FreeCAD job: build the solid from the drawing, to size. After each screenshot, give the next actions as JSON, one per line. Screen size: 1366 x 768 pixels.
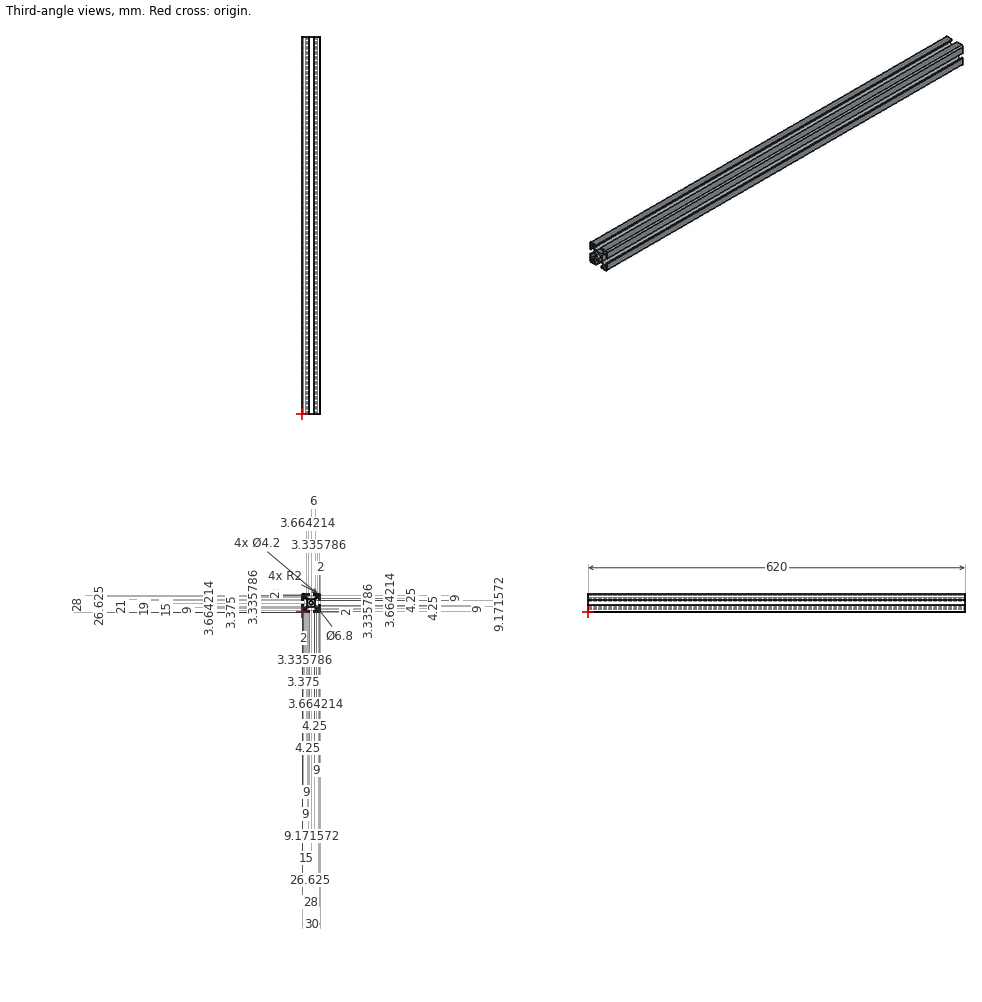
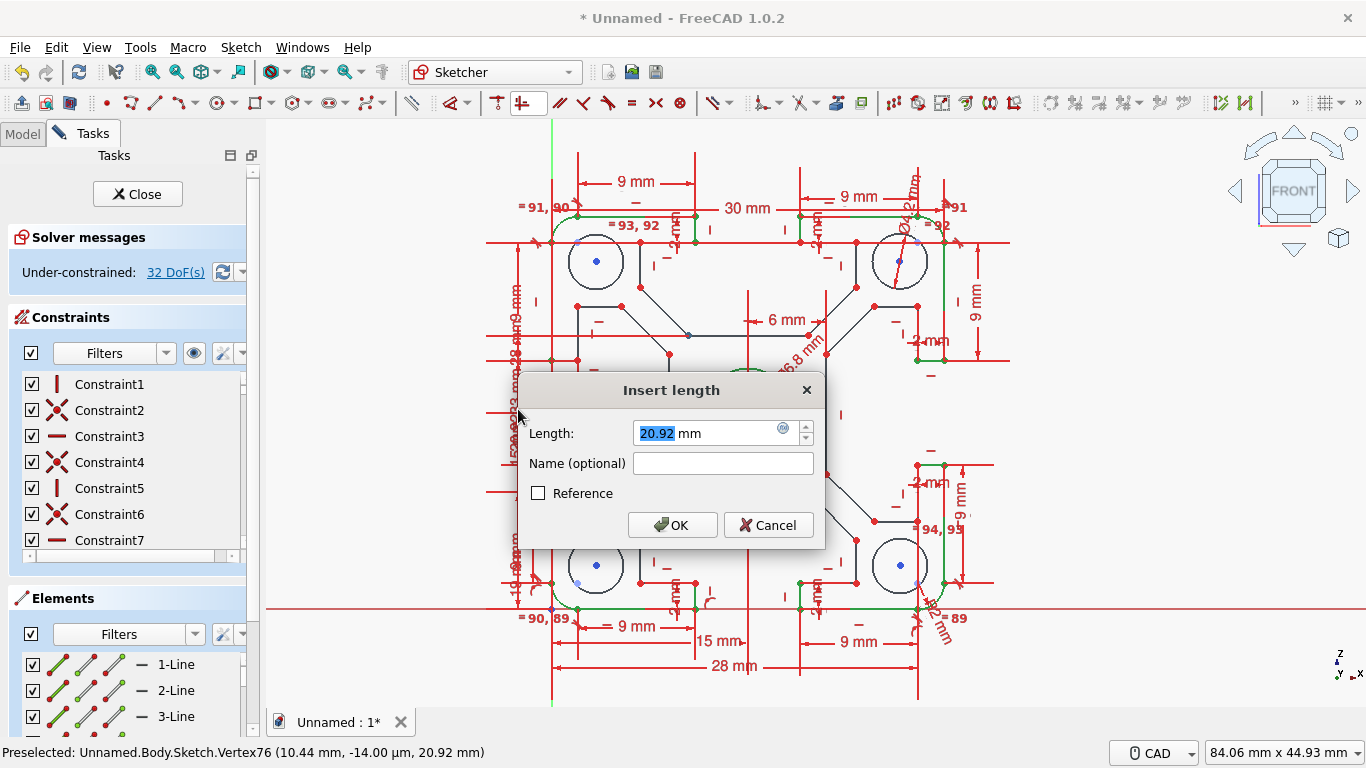
{"action": "type", "text": "21"}
{"action": "key", "text": "Return"}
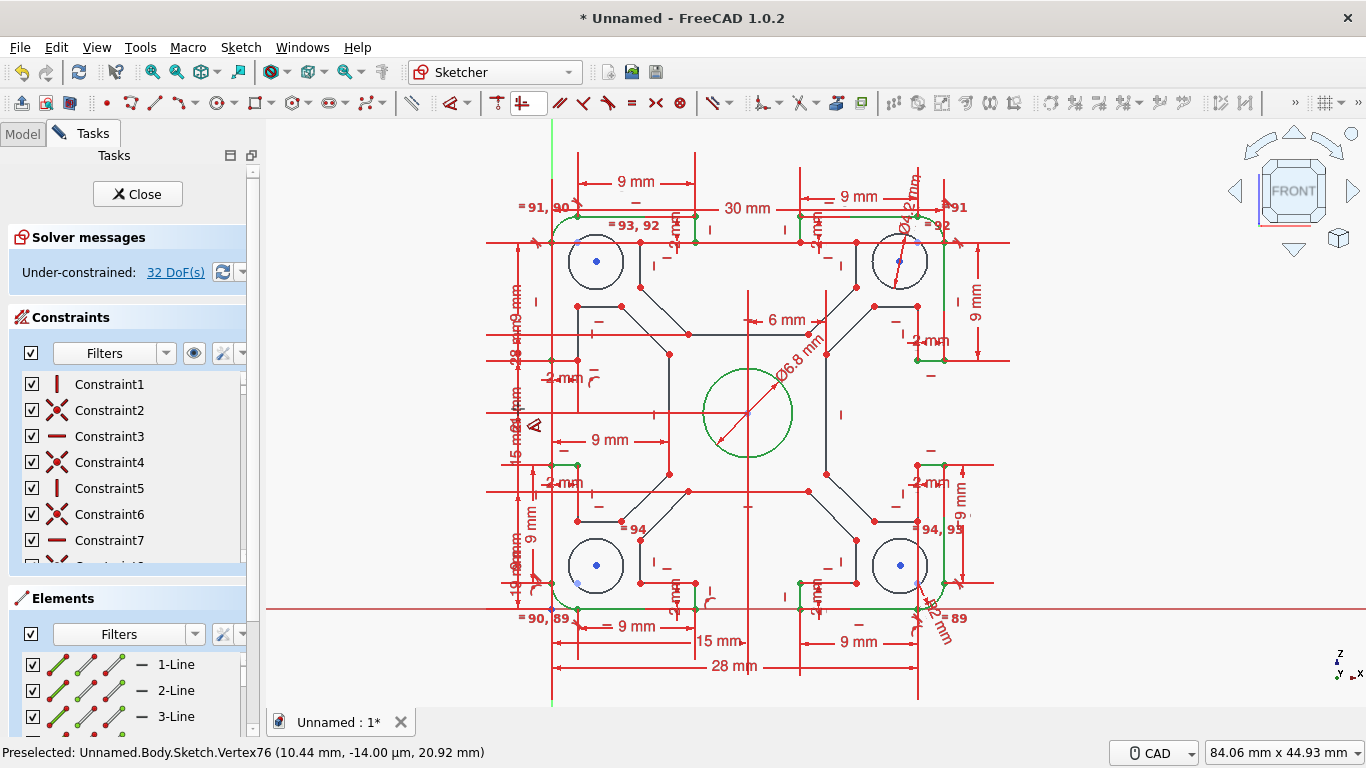
{"action": "left_click", "coordinate": [918, 344]}
{"action": "left_click", "coordinate": [884, 321]}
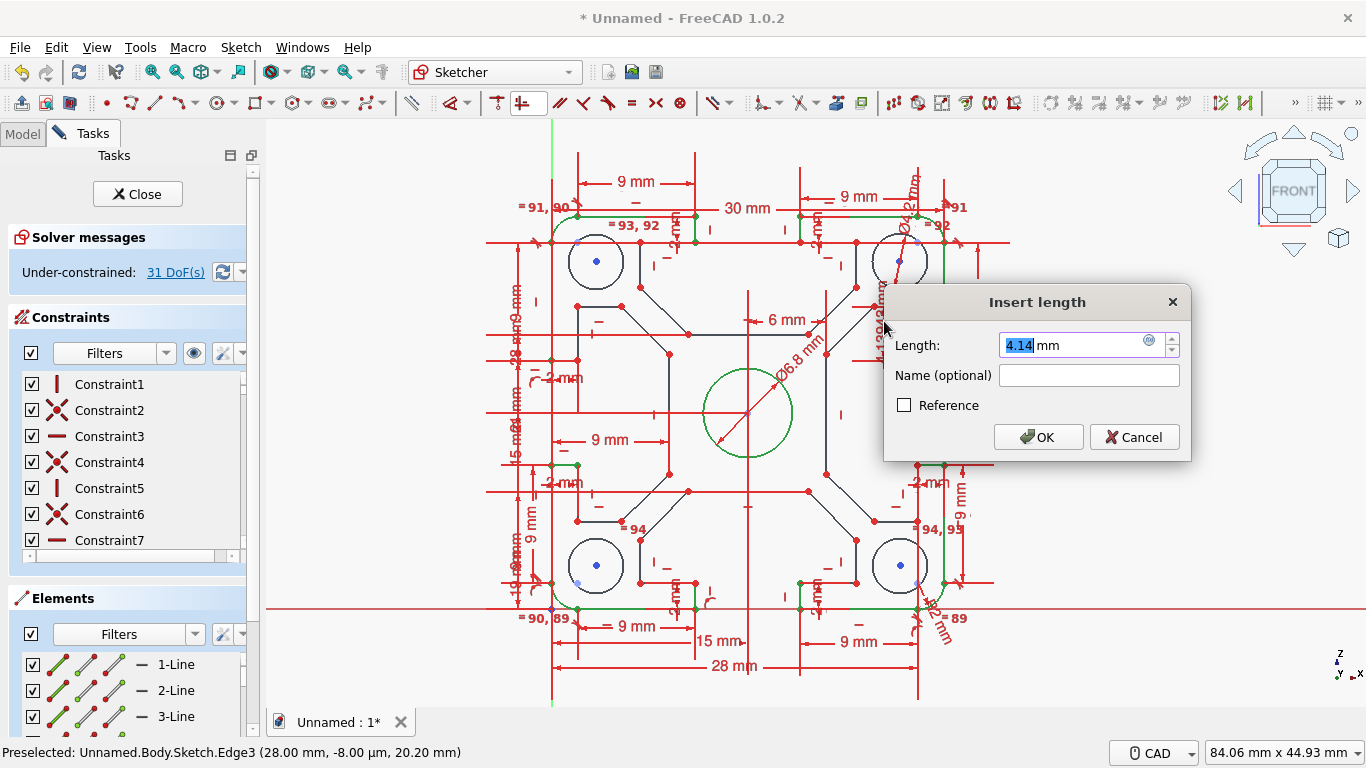
{"action": "type", "text": "4.25"}
{"action": "key", "text": "Return"}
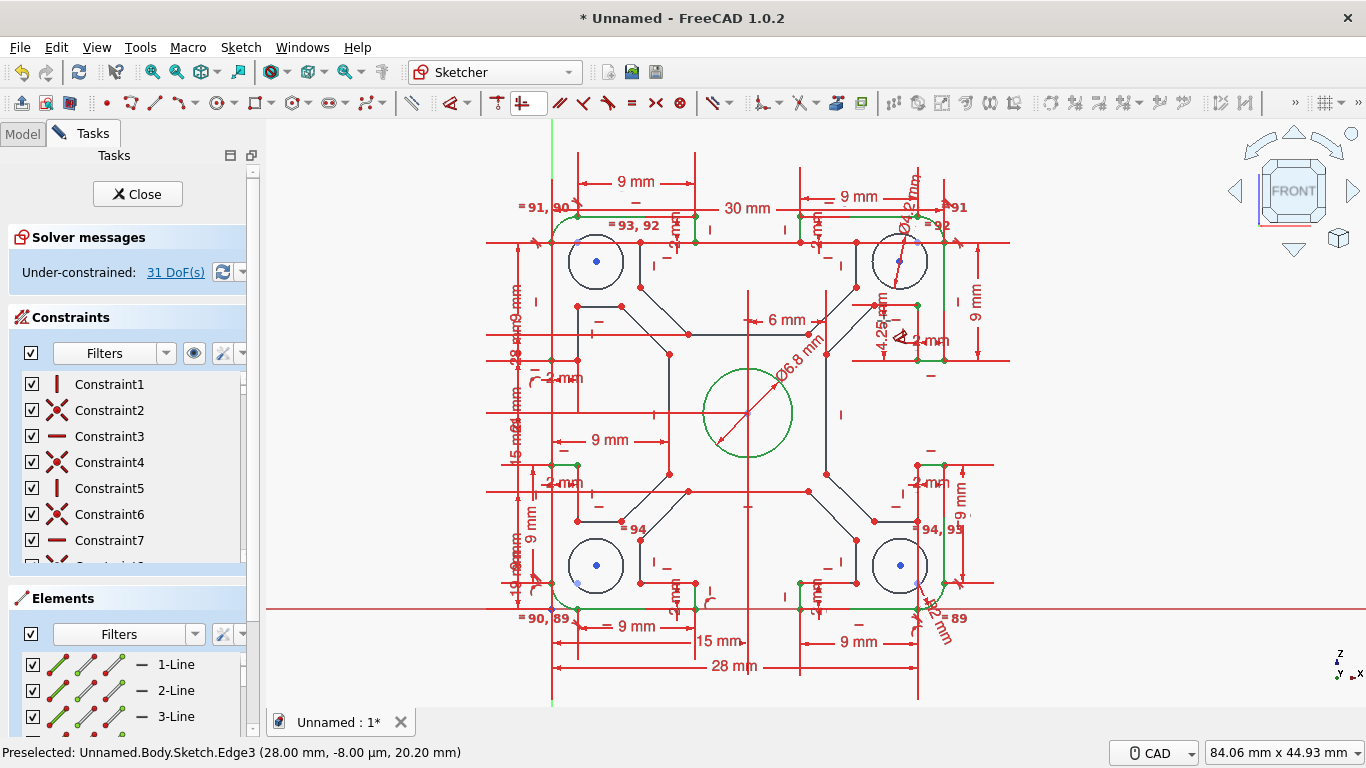
{"action": "left_click", "coordinate": [918, 505]}
{"action": "left_click", "coordinate": [884, 506]}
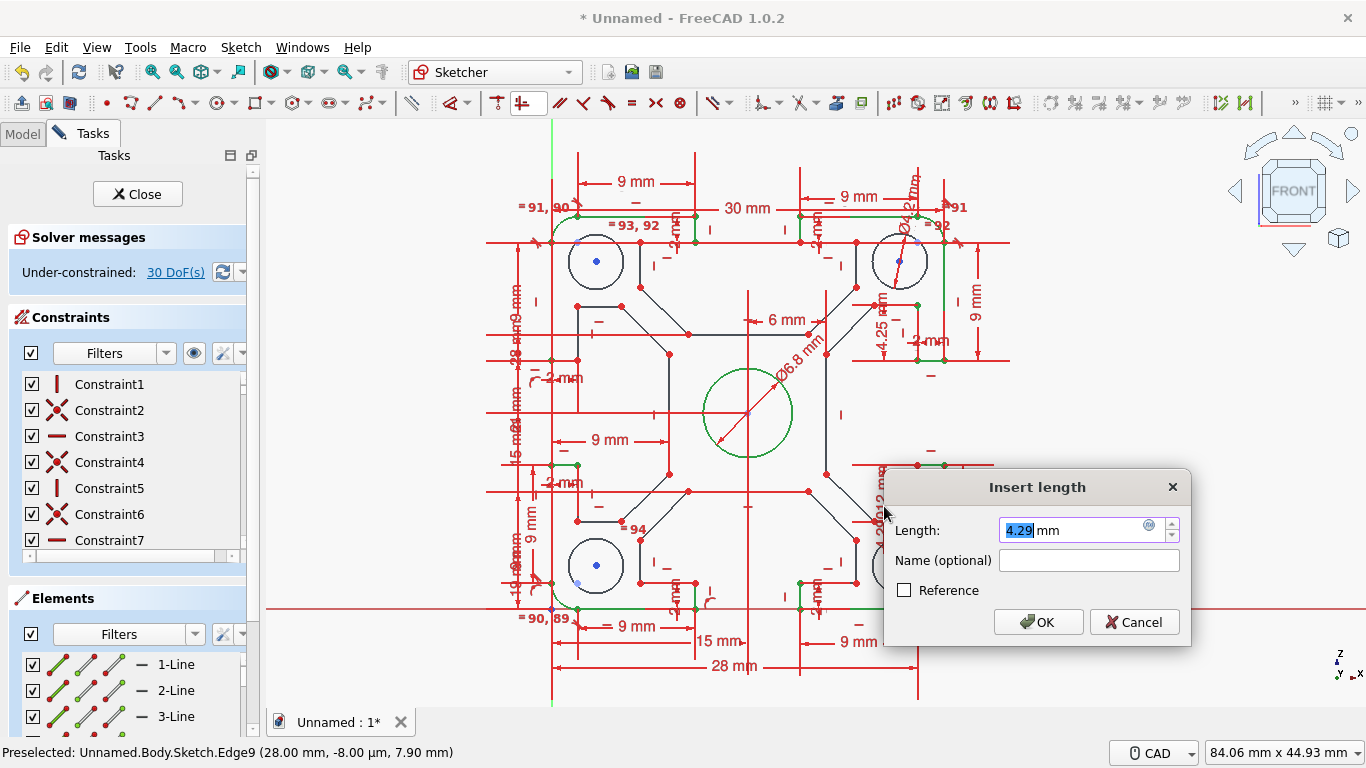
{"action": "type", "text": "4.25"}
{"action": "key", "text": "Return"}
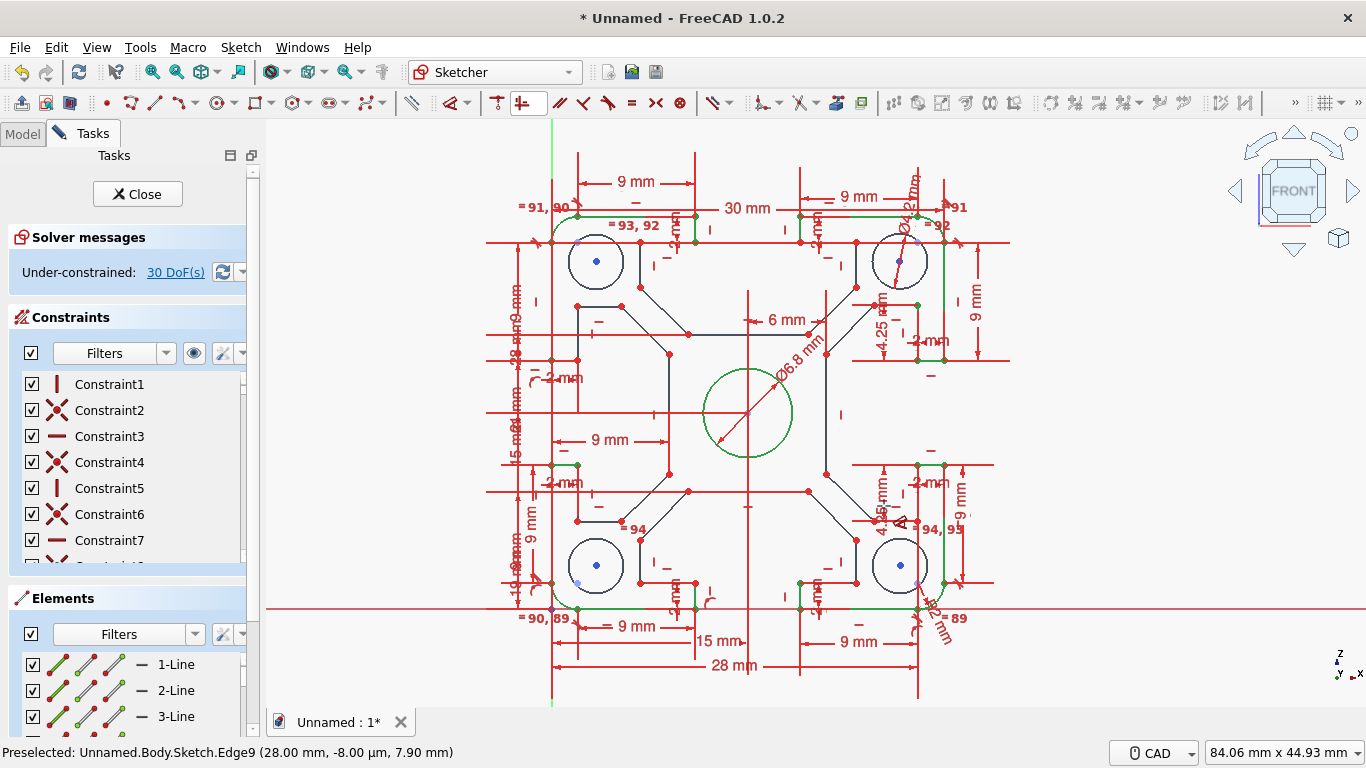
{"action": "left_click", "coordinate": [817, 583]}
{"action": "left_click", "coordinate": [828, 549]}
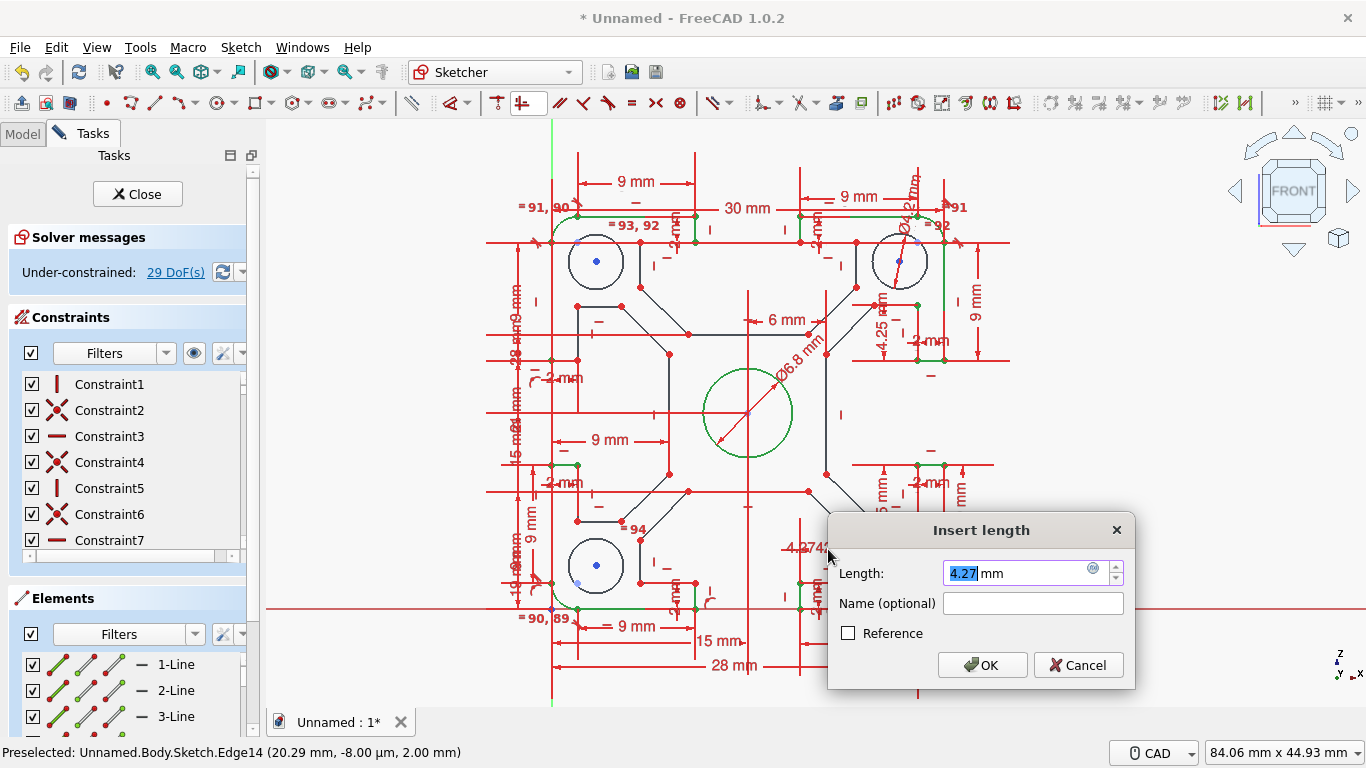
{"action": "type", "text": "4.25"}
{"action": "key", "text": "Return"}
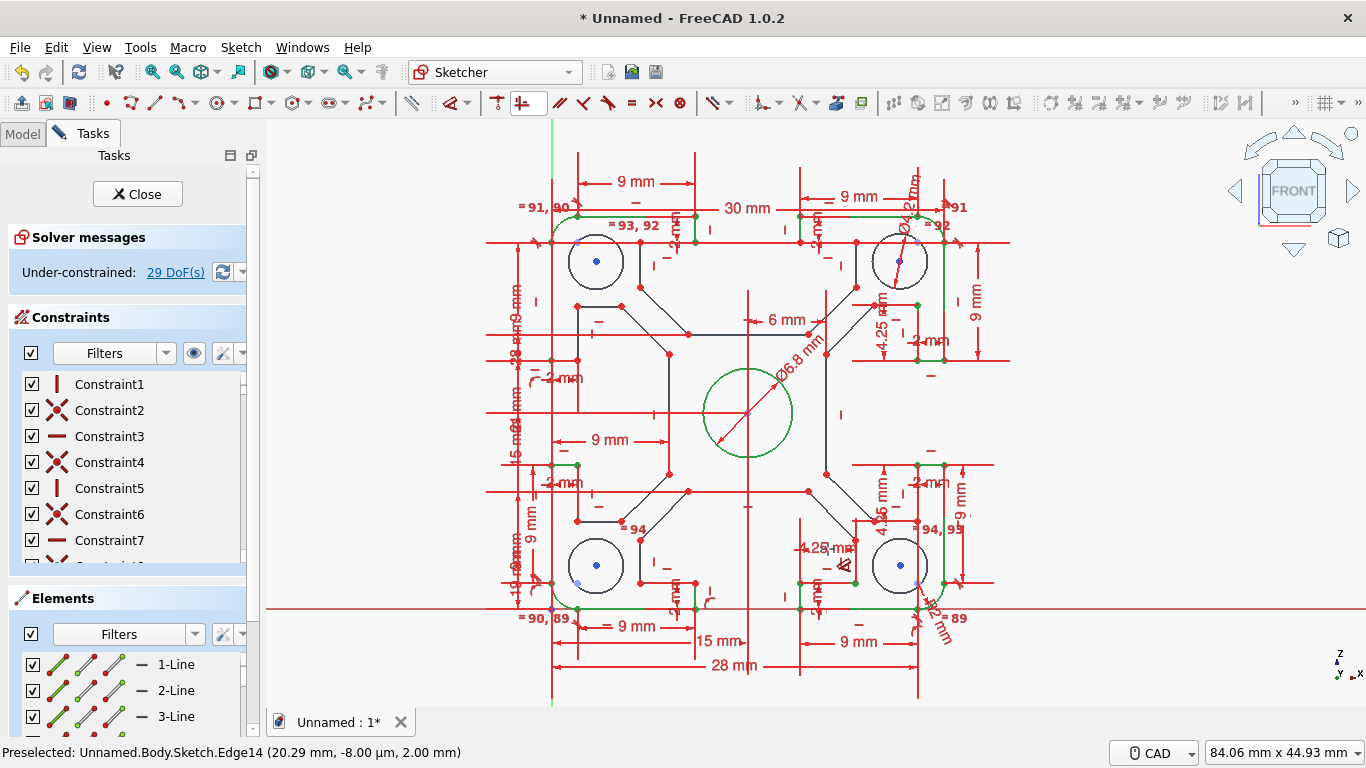
{"action": "left_click", "coordinate": [657, 583]}
{"action": "left_click", "coordinate": [668, 549]}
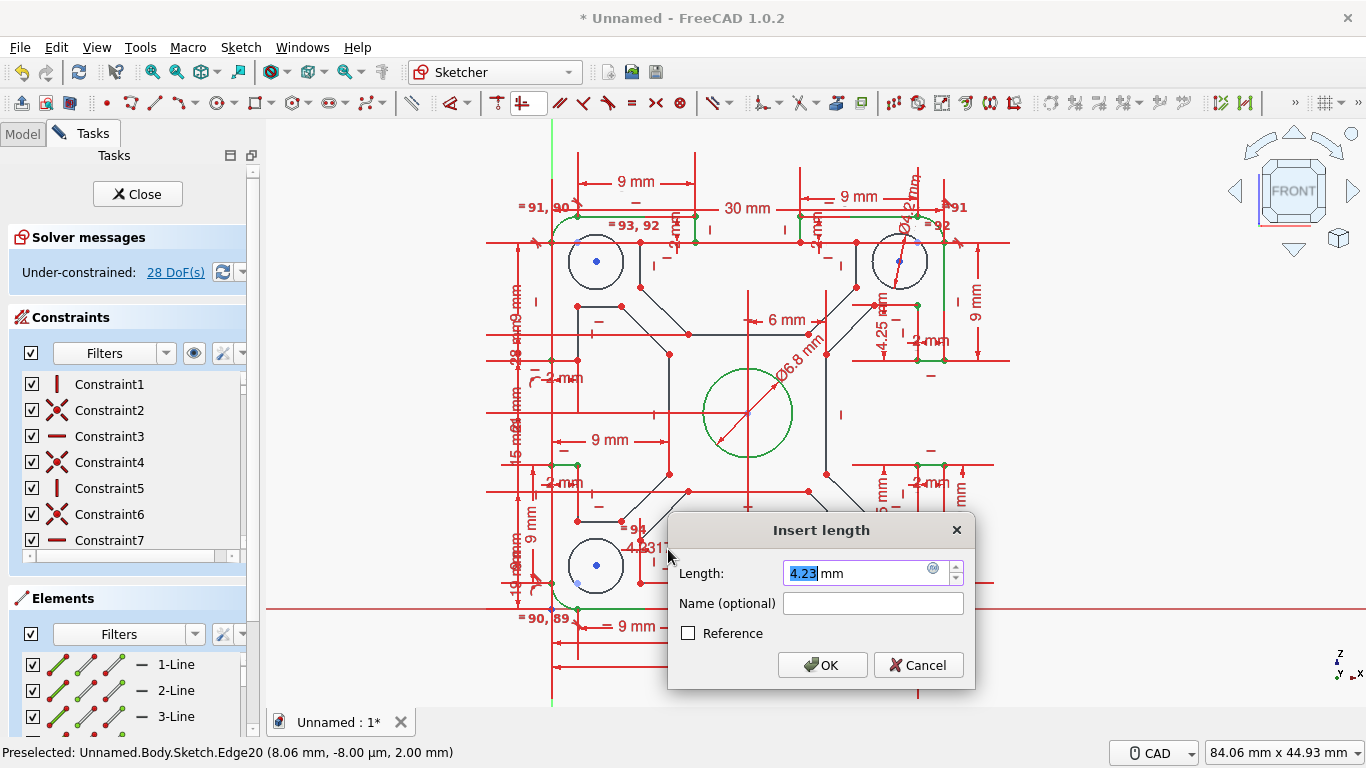
{"action": "type", "text": "4.25"}
{"action": "key", "text": "Return"}